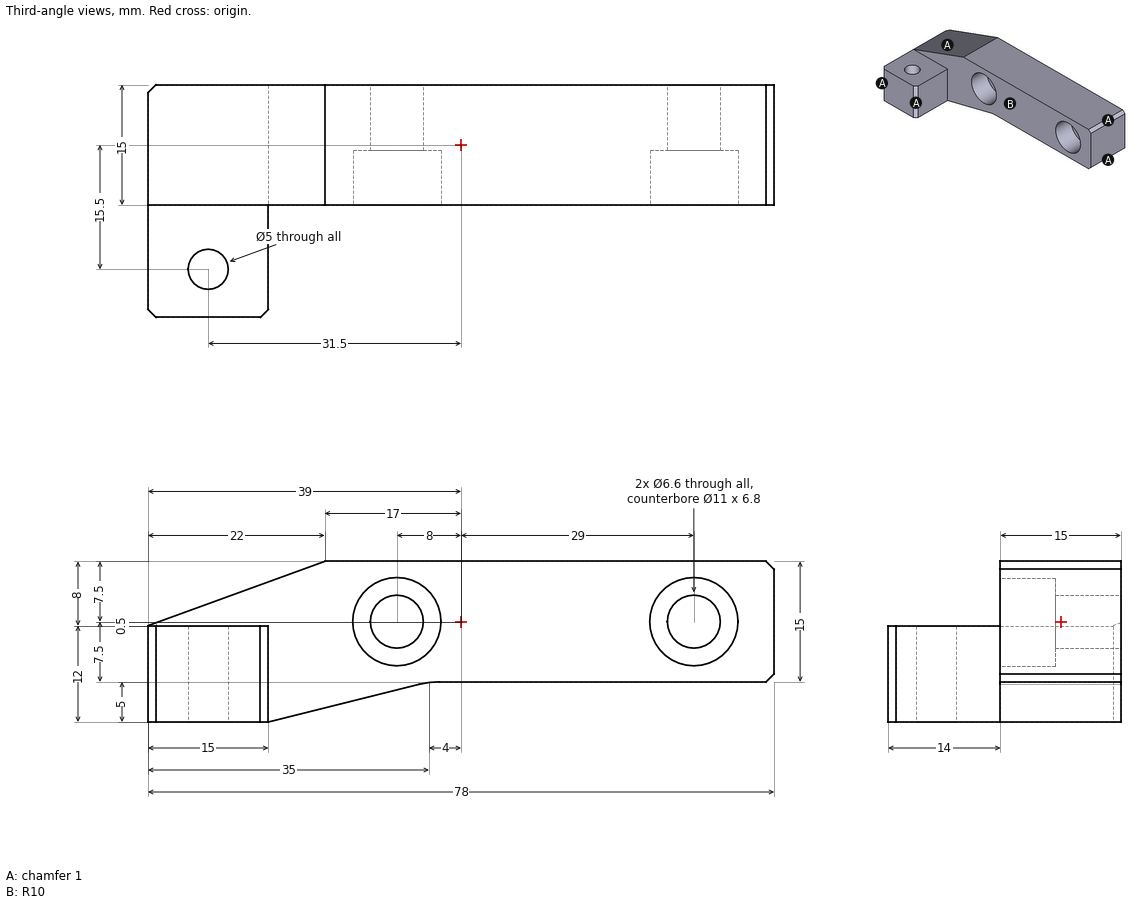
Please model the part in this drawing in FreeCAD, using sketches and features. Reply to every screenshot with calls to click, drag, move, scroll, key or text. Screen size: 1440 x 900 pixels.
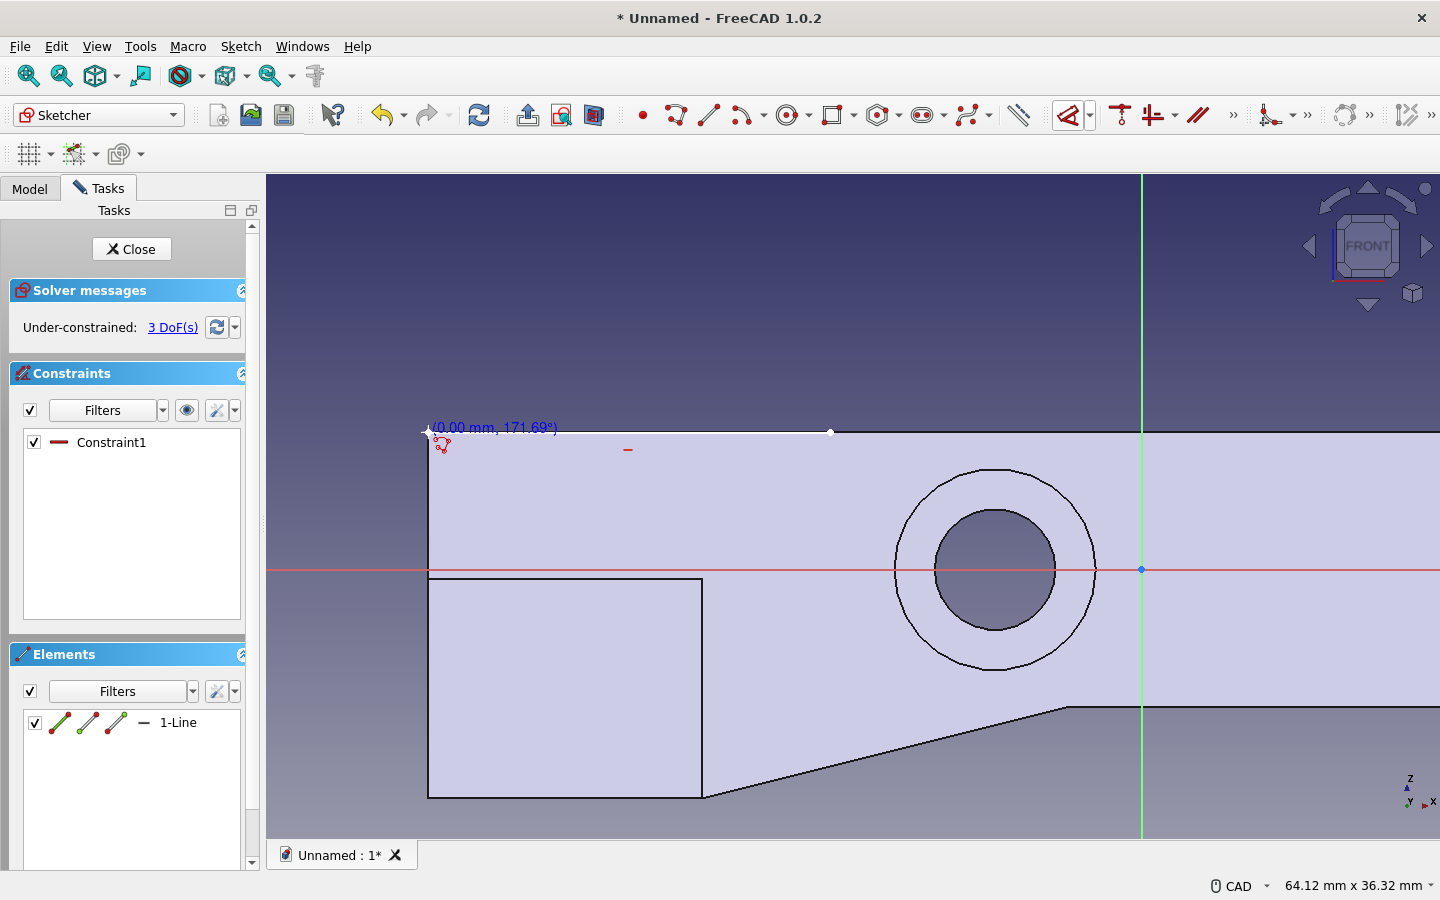
scroll(428, 579, up, 3)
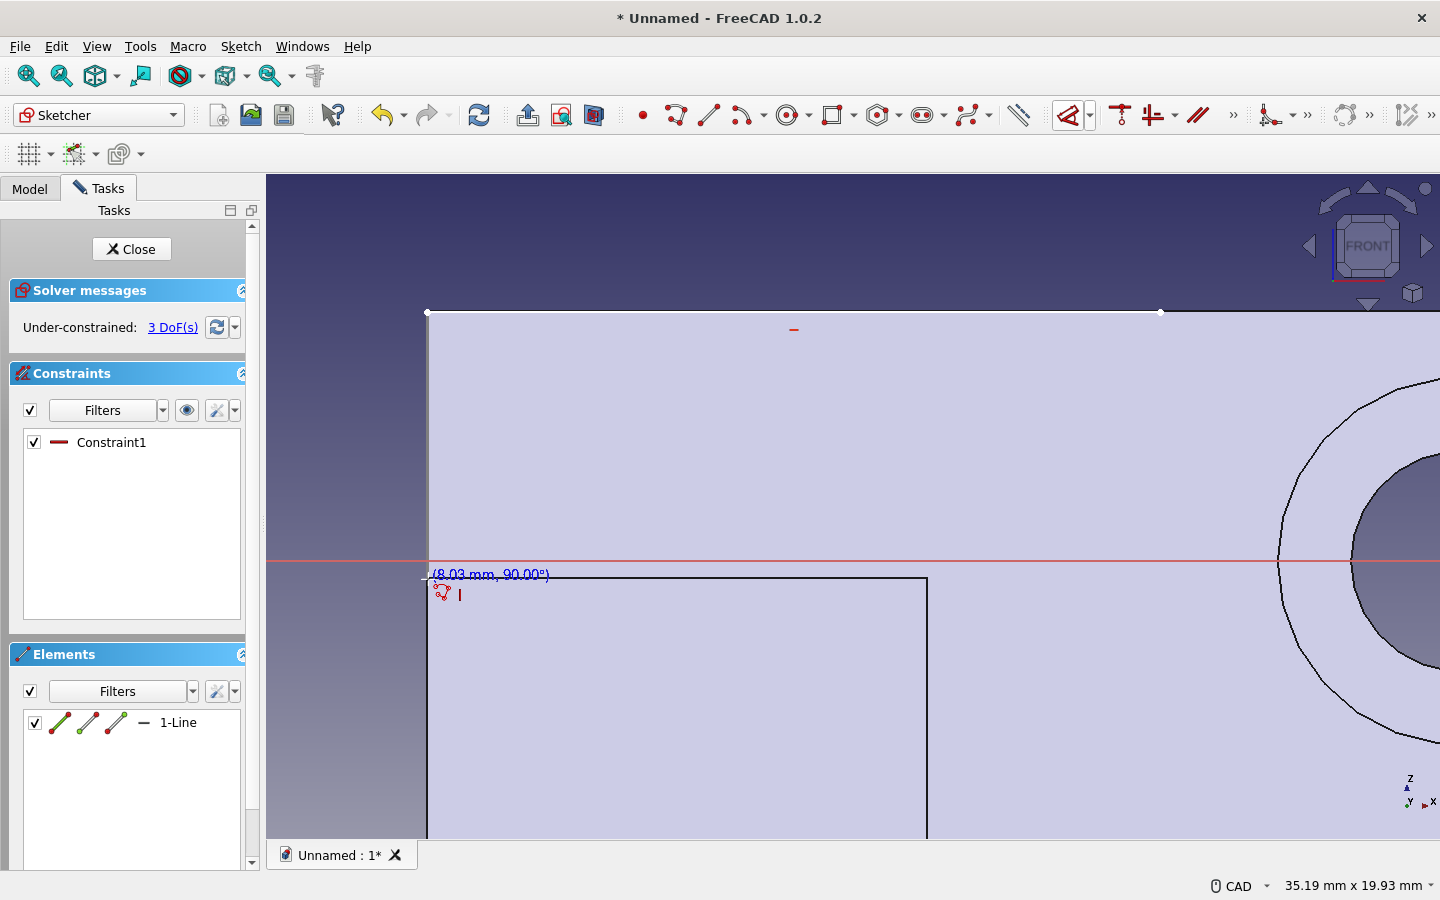
click(428, 578)
click(1160, 312)
key(Escape)
key(Escape)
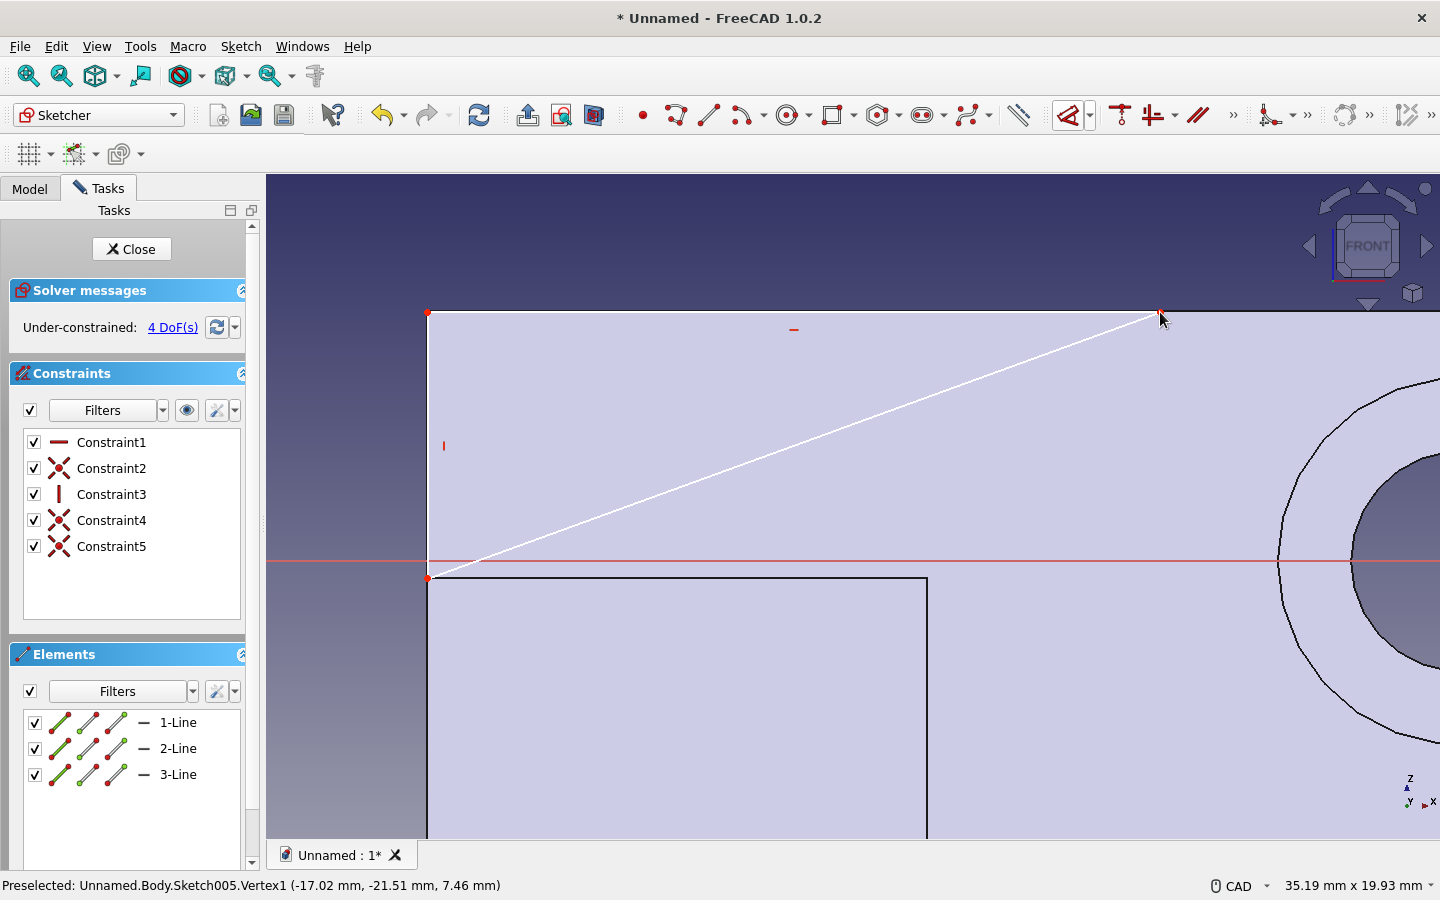
click(428, 392)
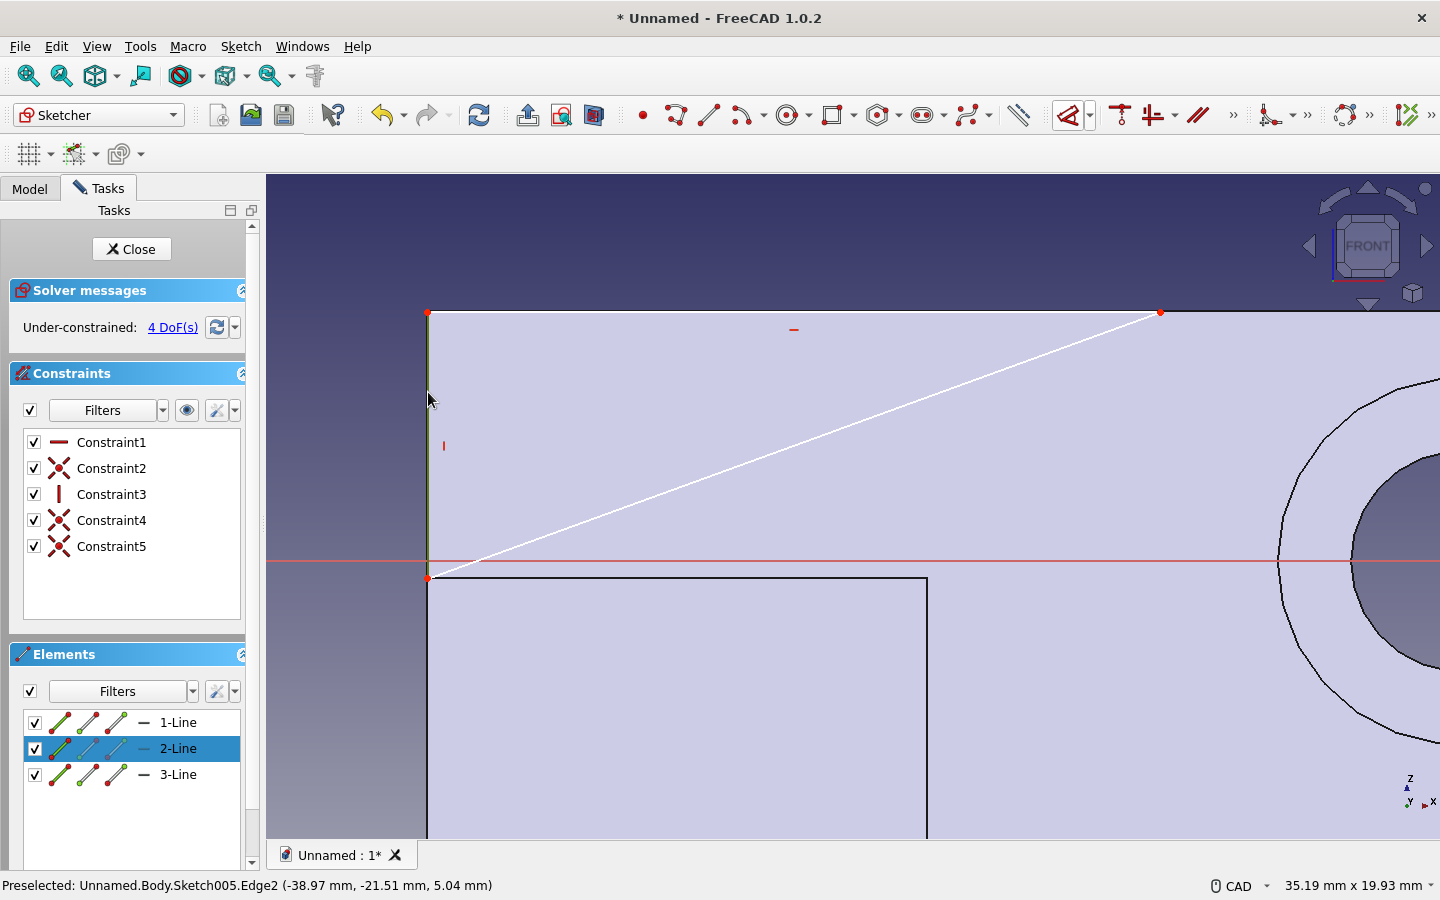
click(1090, 116)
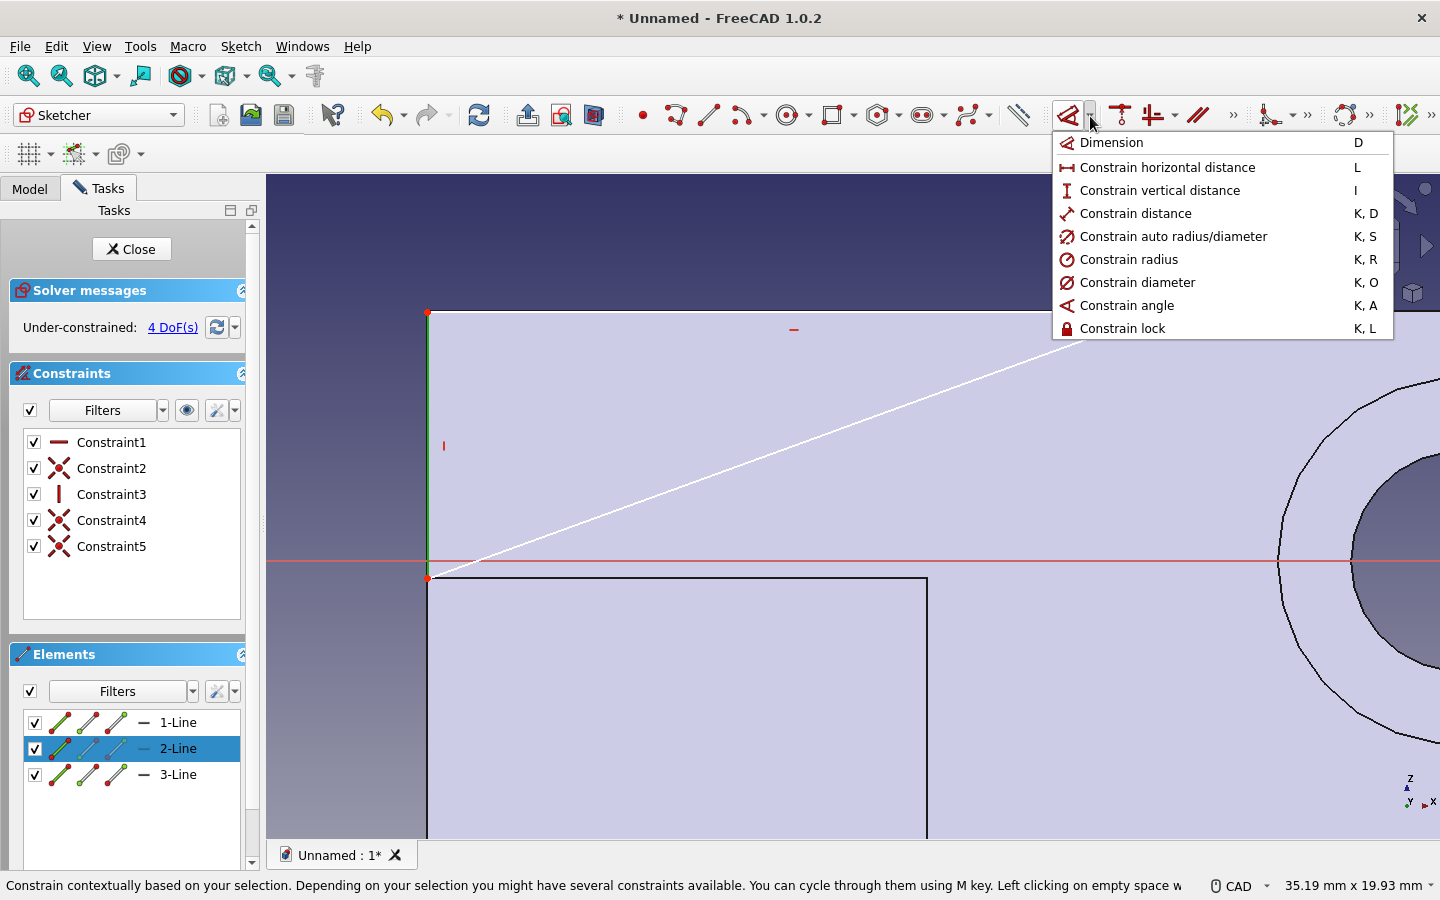
click(1223, 190)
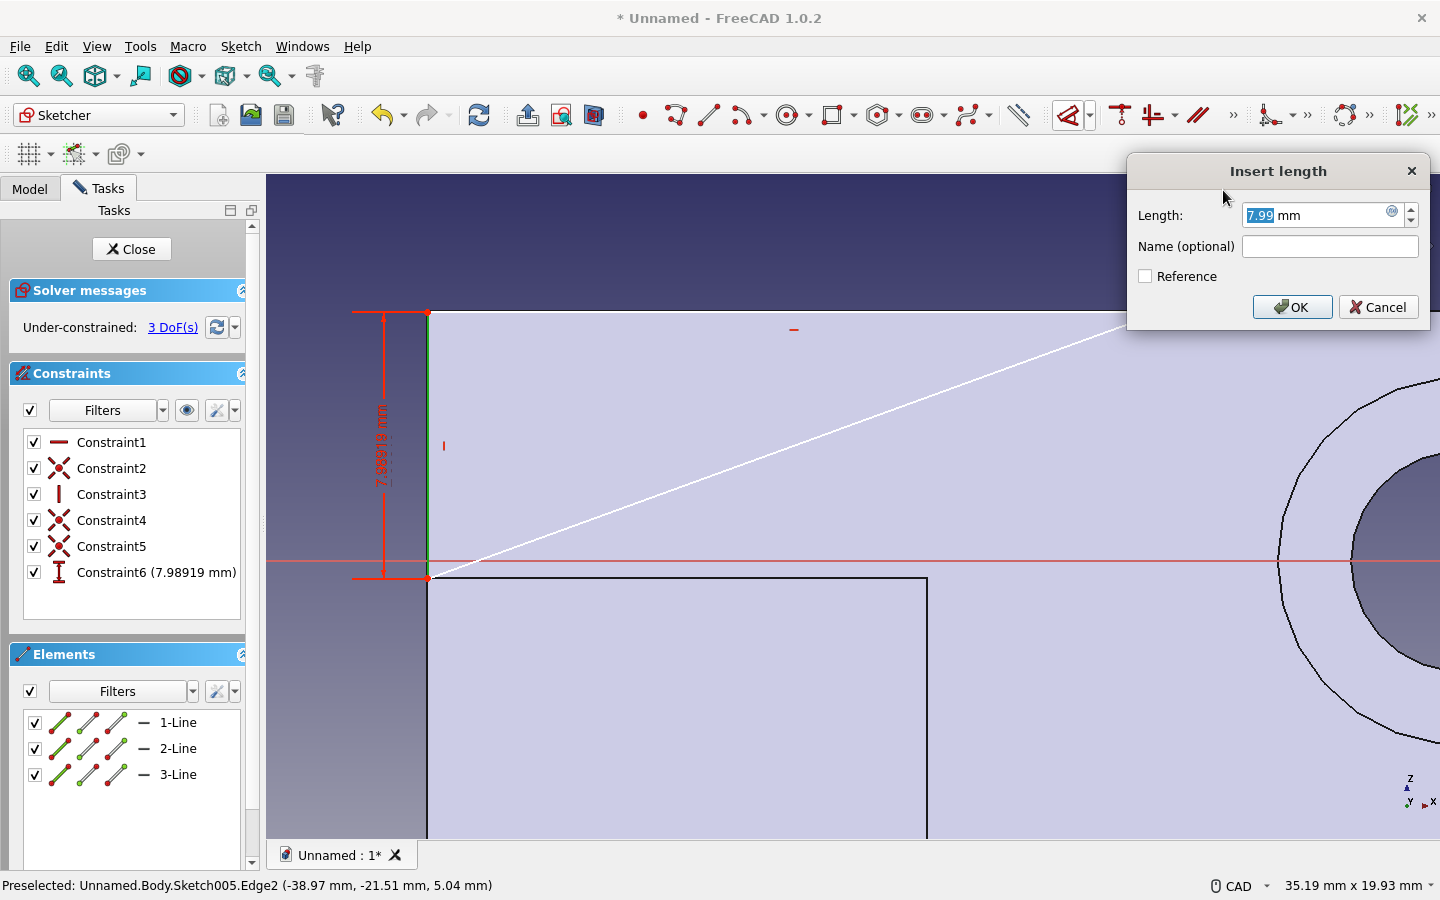
text(8)
key(Return)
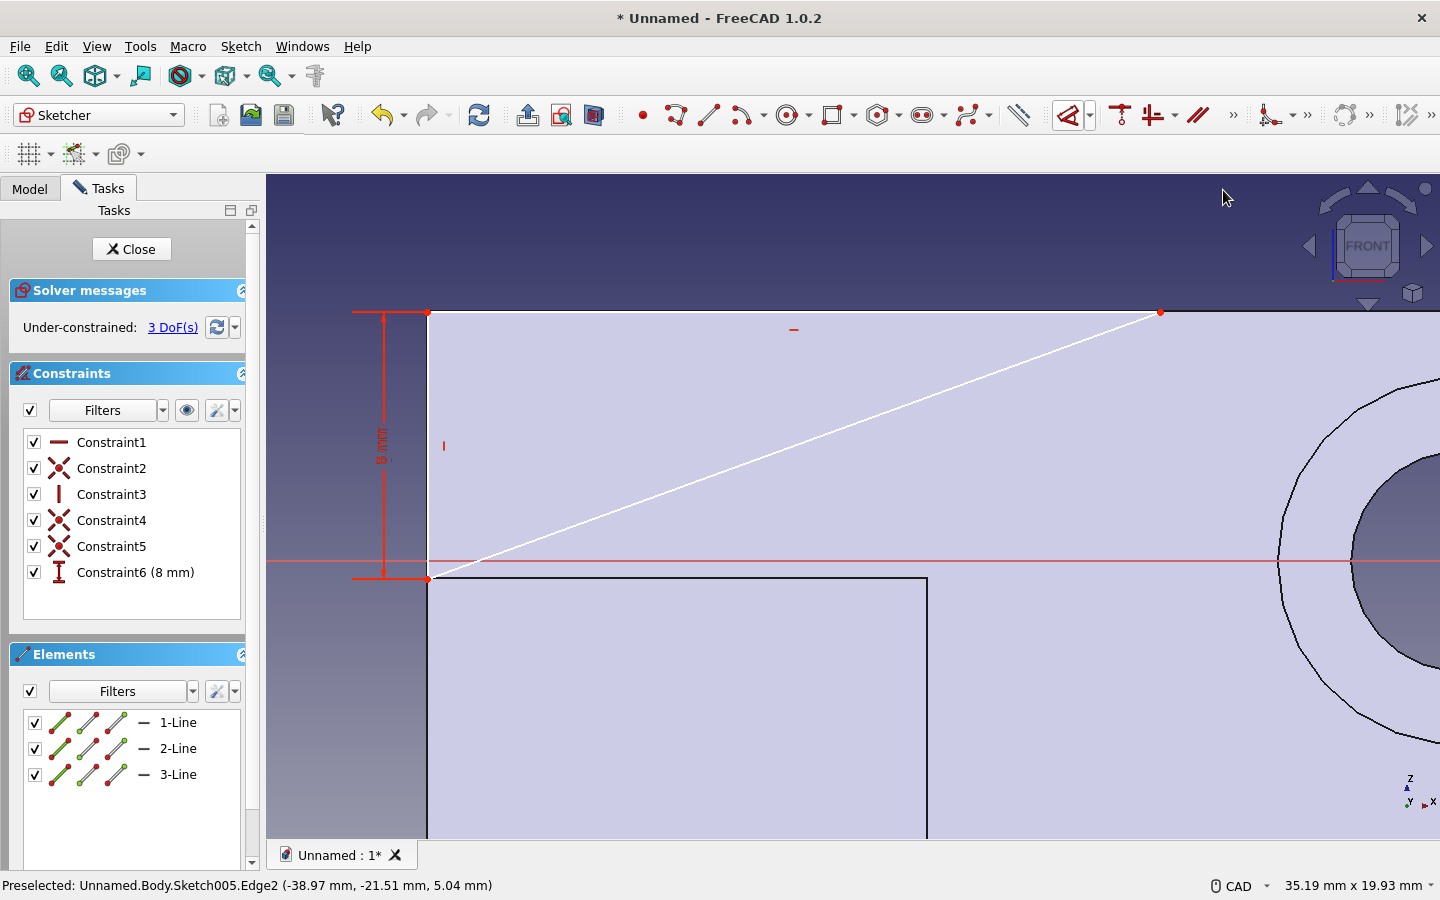
click(941, 312)